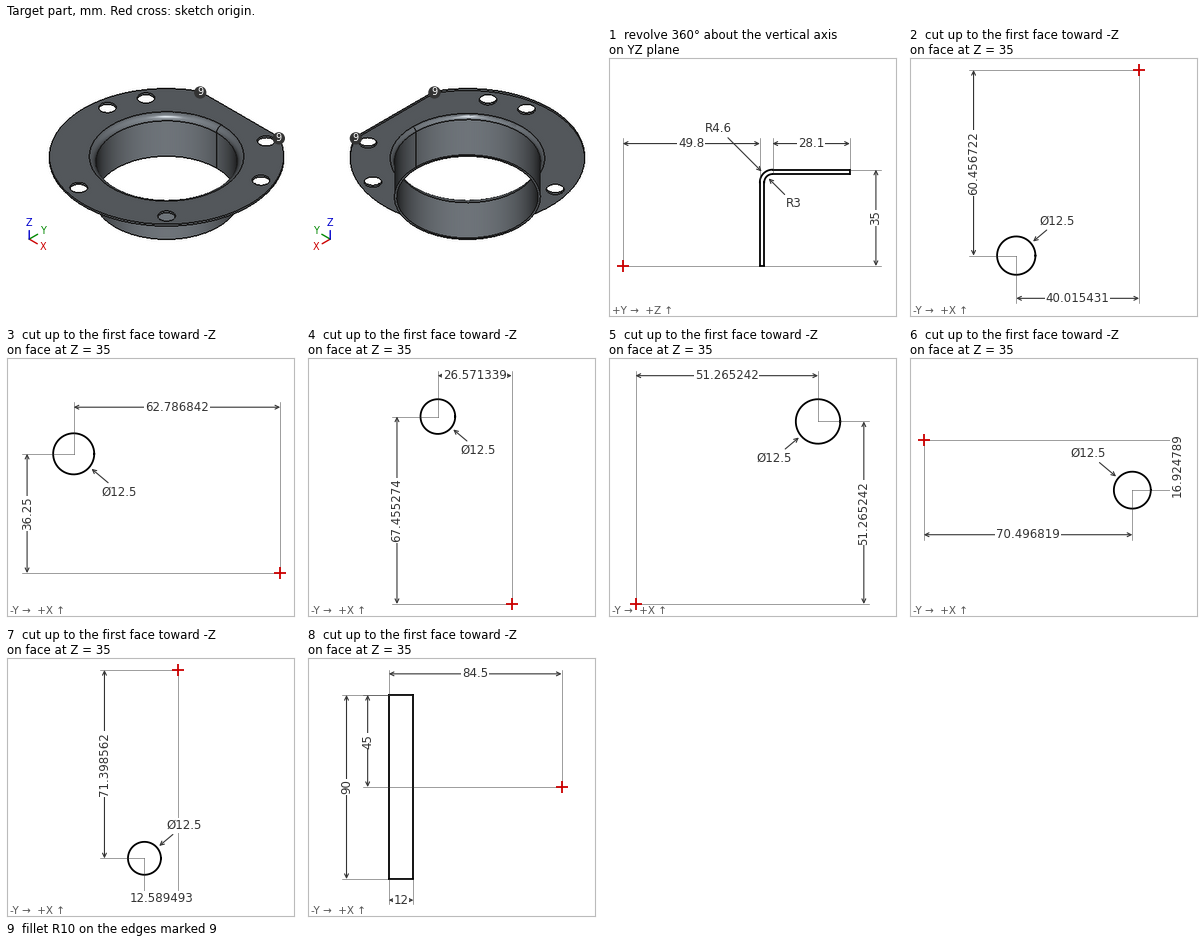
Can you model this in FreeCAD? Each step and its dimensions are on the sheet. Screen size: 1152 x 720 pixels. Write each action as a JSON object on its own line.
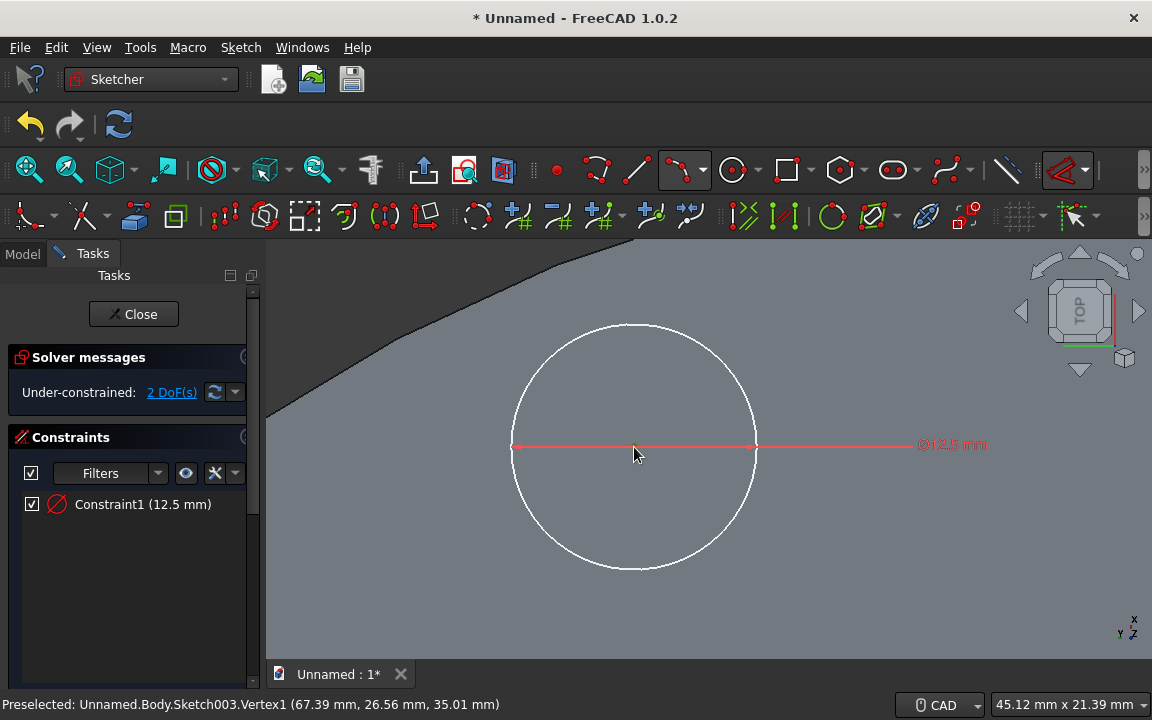
{"action": "key", "text": "l"}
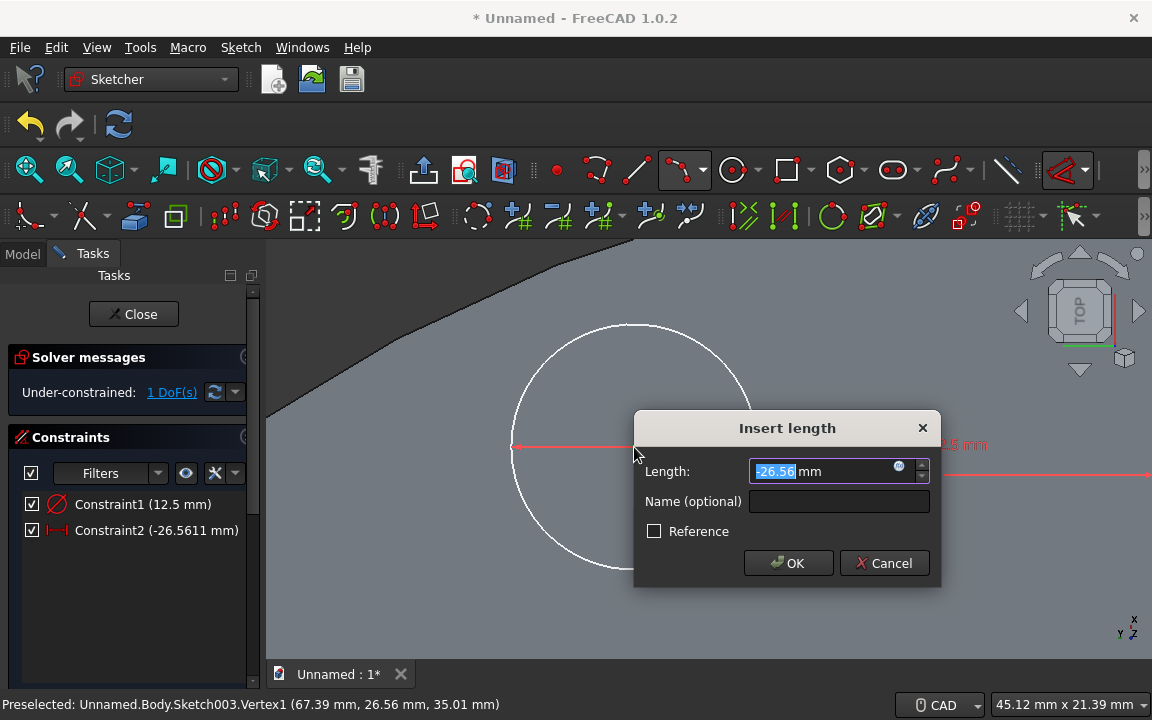
{"action": "type", "text": "-26.571339"}
{"action": "key", "text": "Return"}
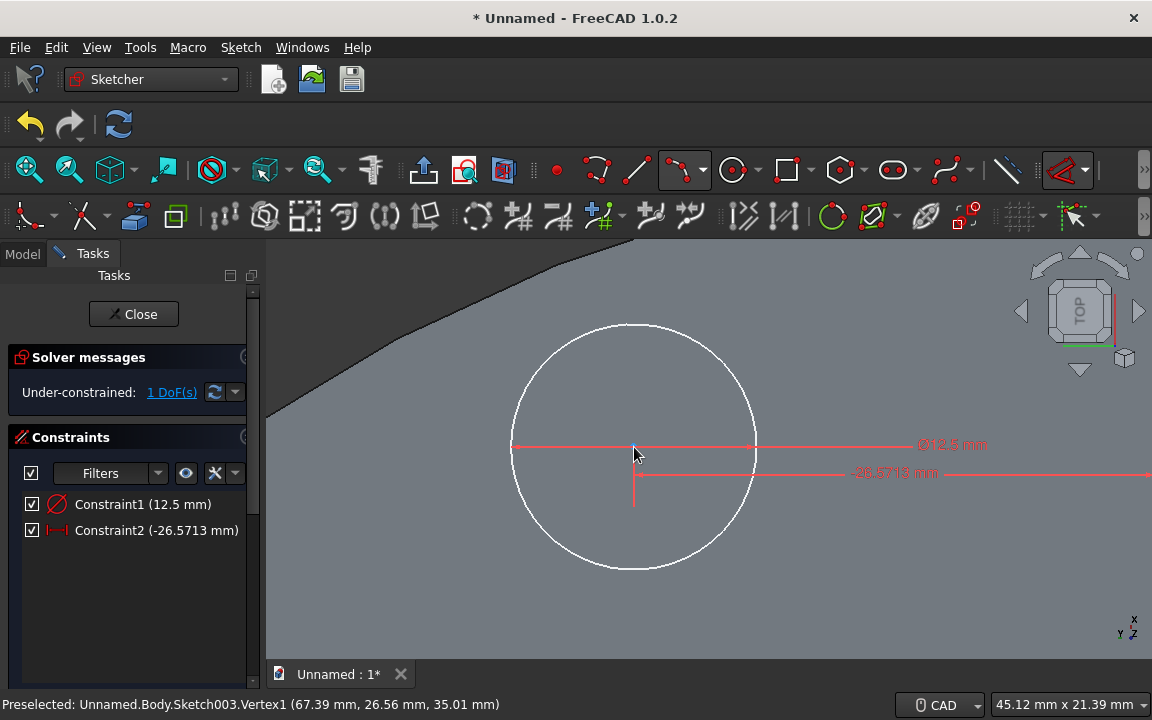
{"action": "left_click", "coordinate": [634, 447]}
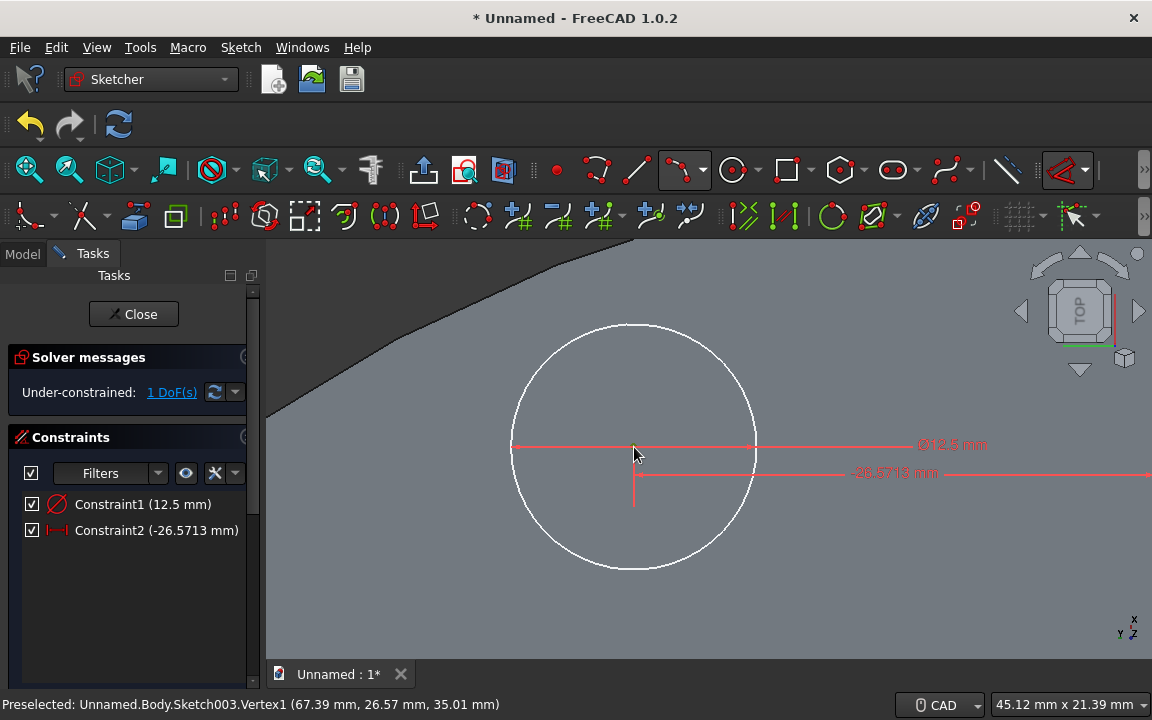
{"action": "key", "text": "i"}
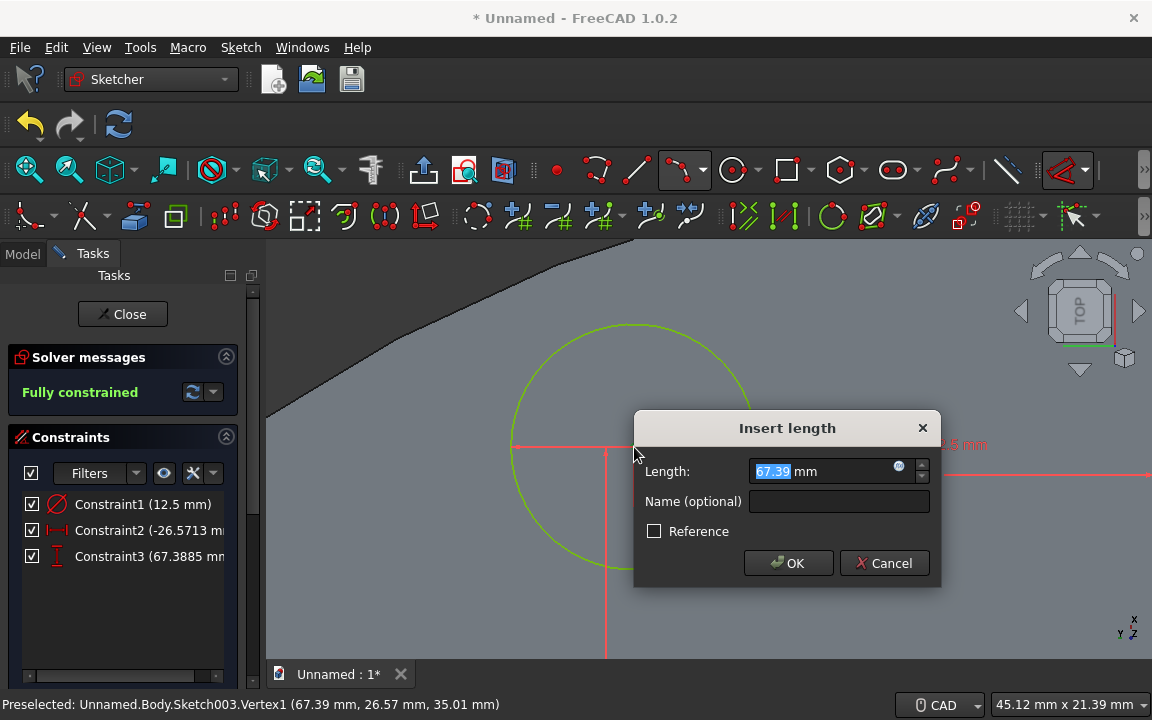
{"action": "type", "text": "67.455274"}
{"action": "key", "text": "Return"}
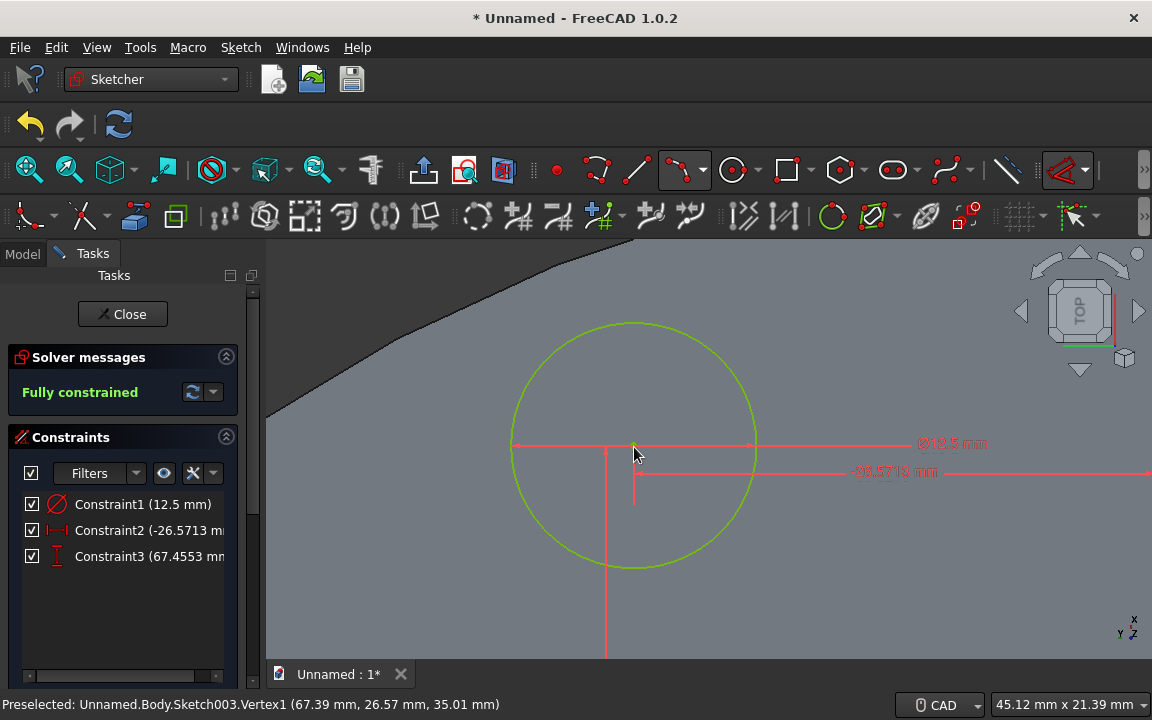
{"action": "left_click", "coordinate": [123, 314]}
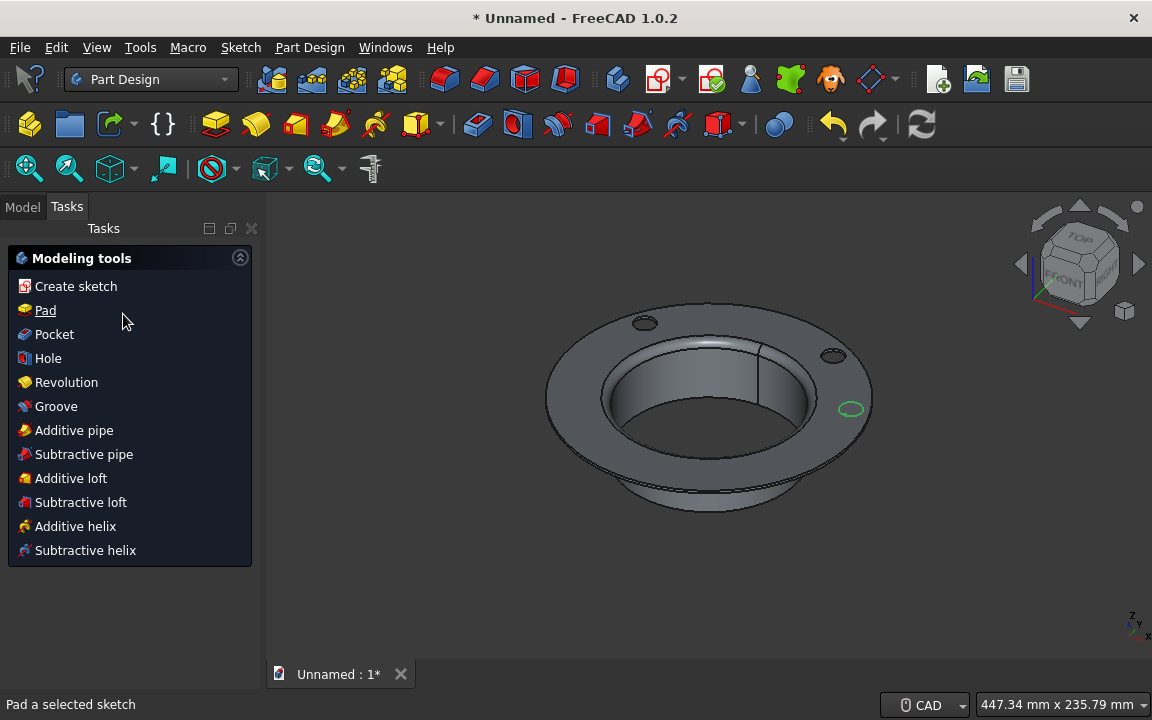
{"action": "left_click", "coordinate": [478, 124]}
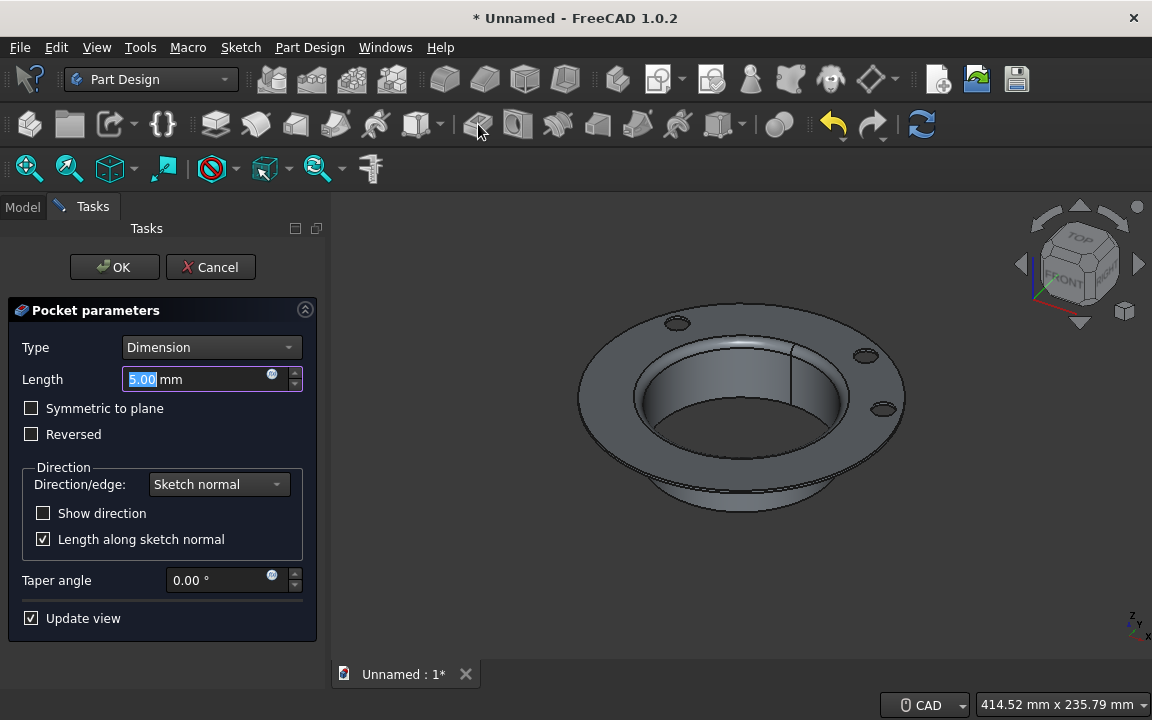
{"action": "left_click", "coordinate": [212, 348]}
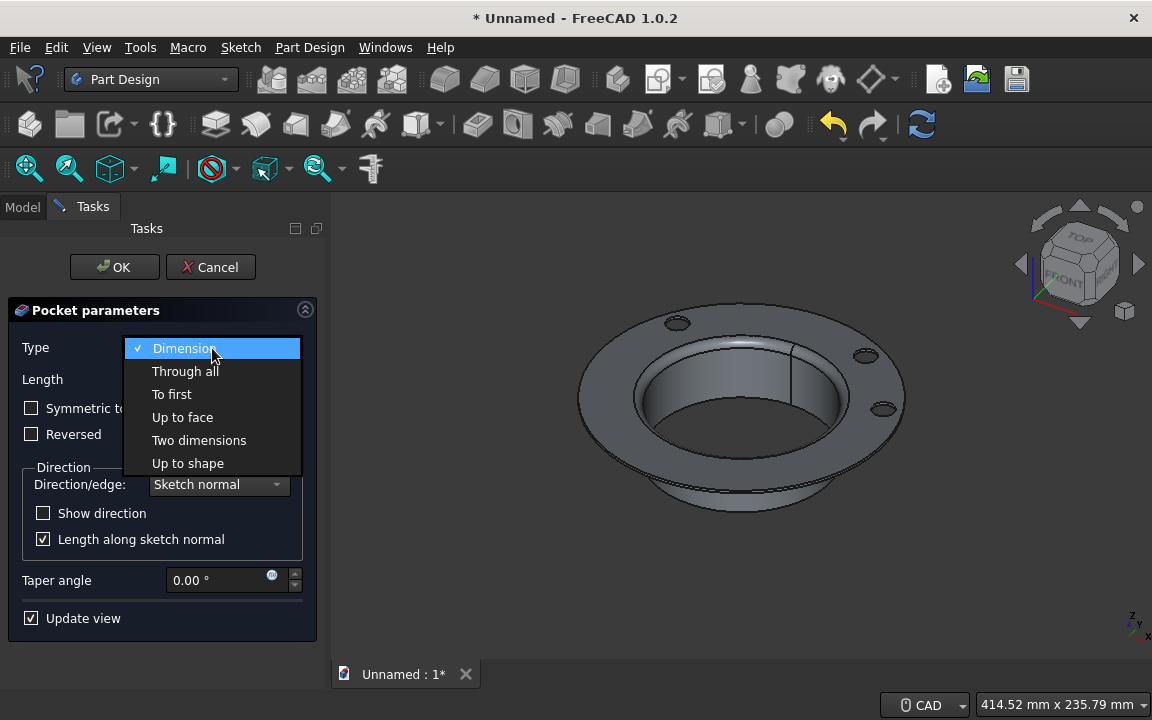
{"action": "left_click", "coordinate": [212, 394]}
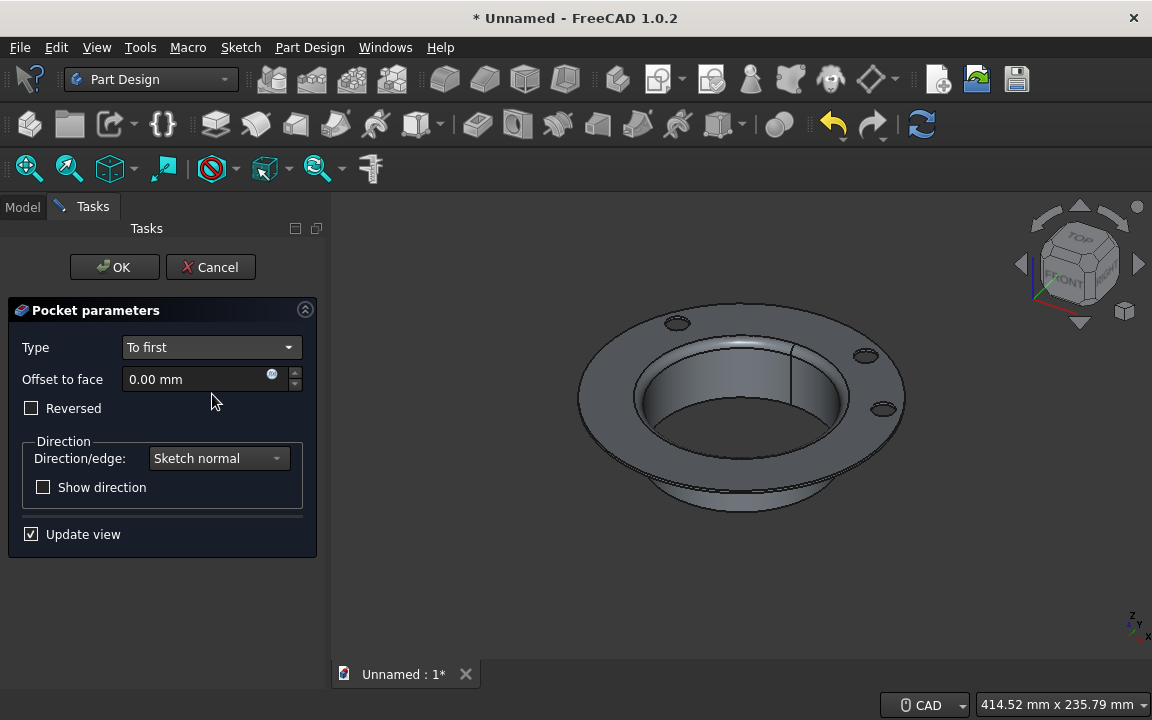
{"action": "left_click", "coordinate": [115, 267]}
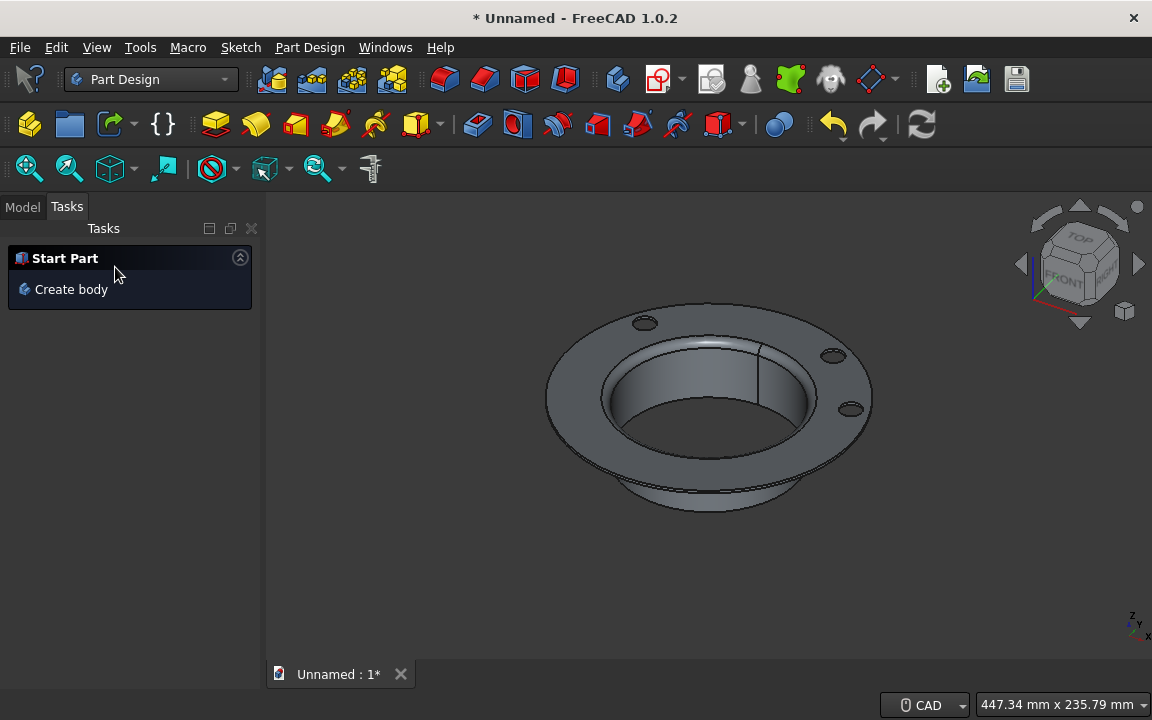
{"action": "left_click", "coordinate": [837, 377]}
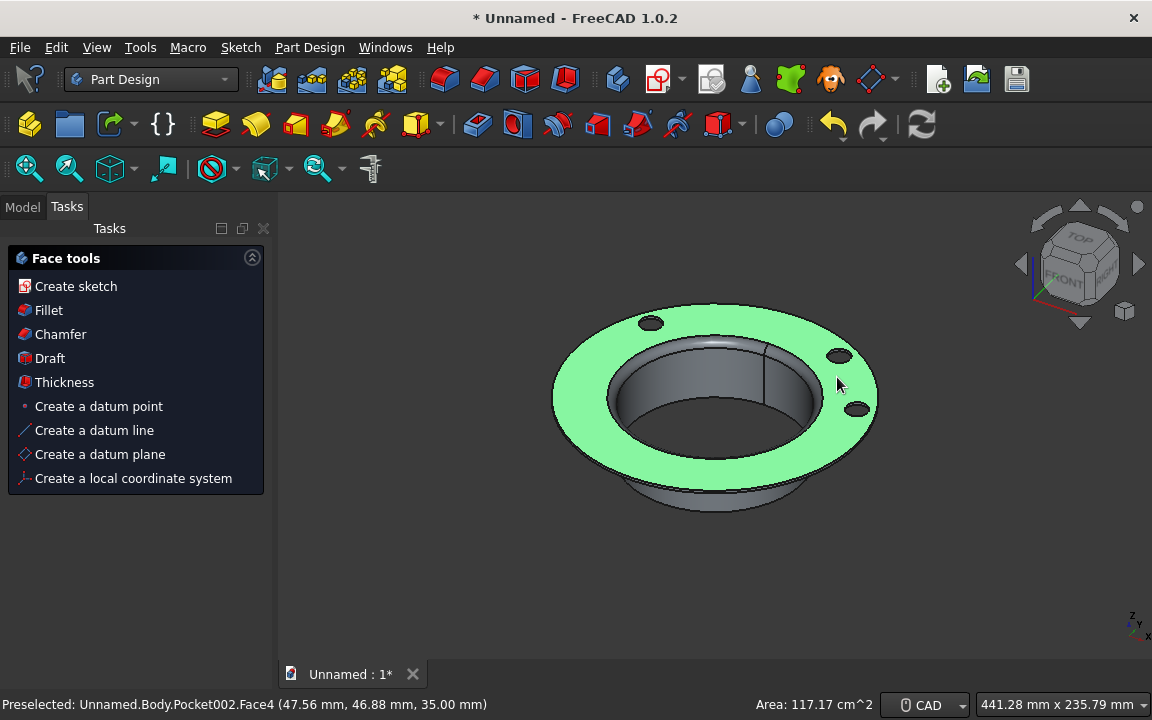
{"action": "left_click", "coordinate": [658, 80]}